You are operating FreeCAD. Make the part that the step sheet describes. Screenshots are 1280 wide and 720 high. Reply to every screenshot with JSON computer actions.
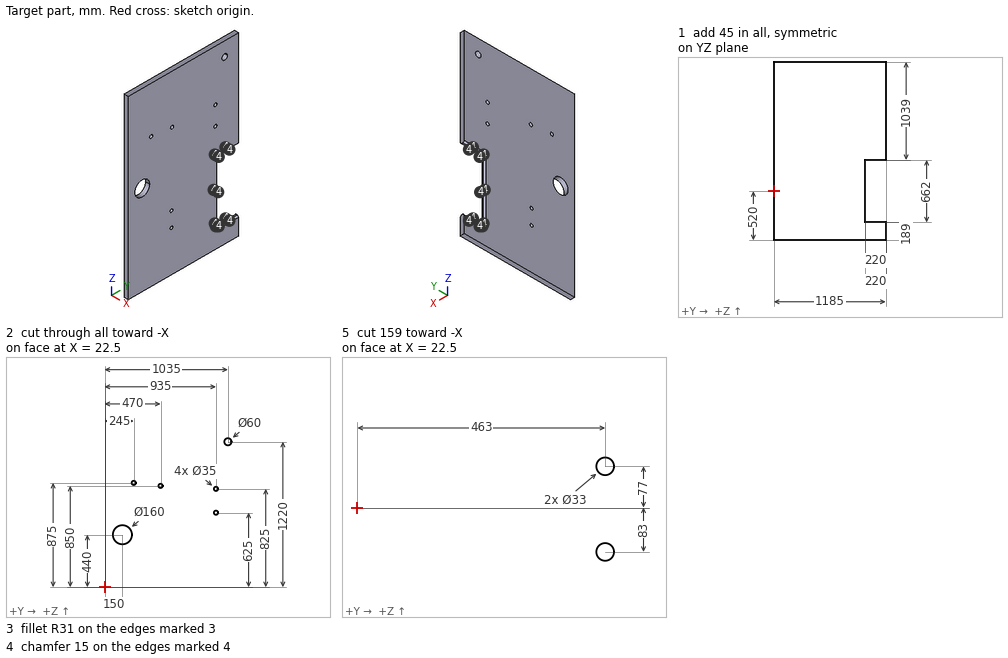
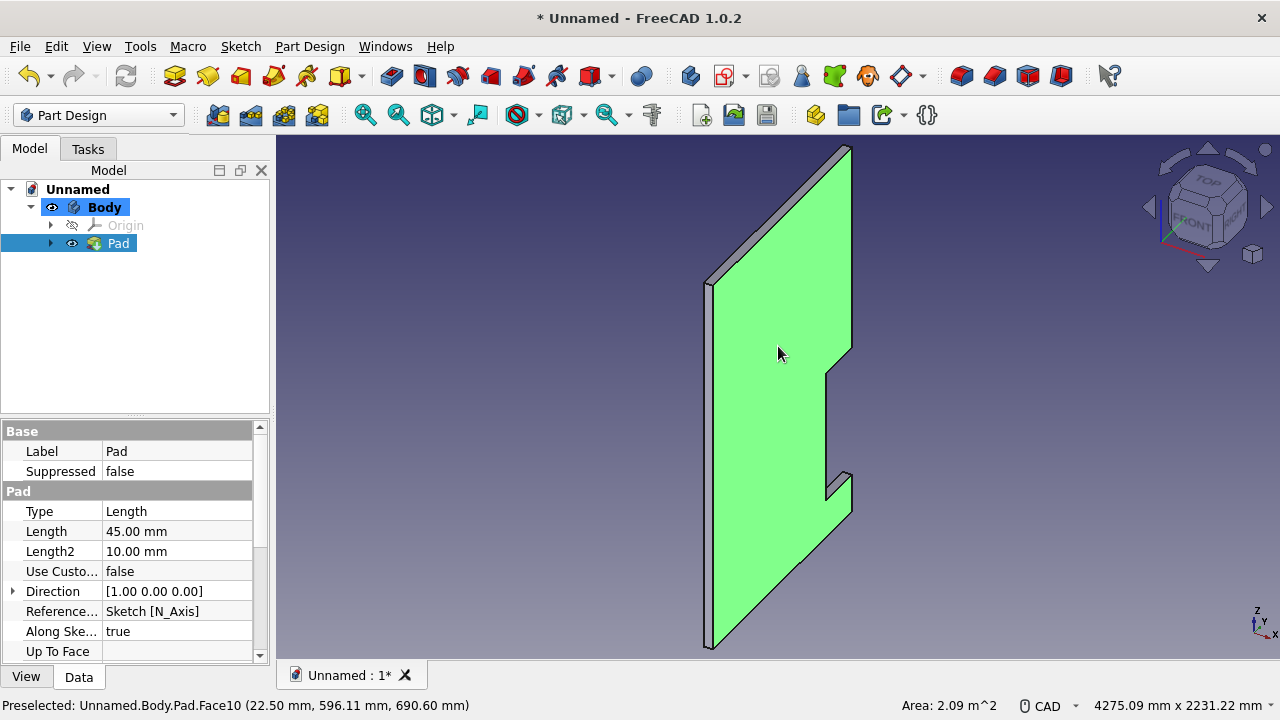
{"action": "left_click", "coordinate": [724, 76]}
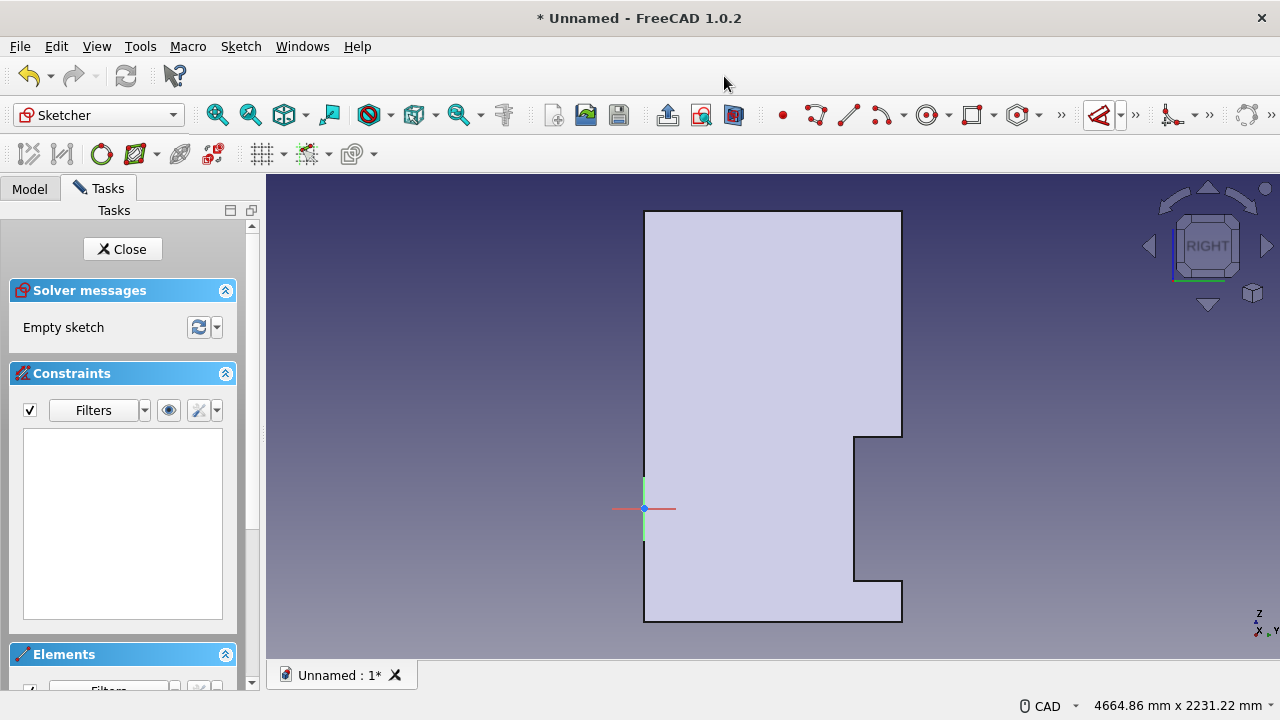
{"action": "left_click", "coordinate": [926, 116]}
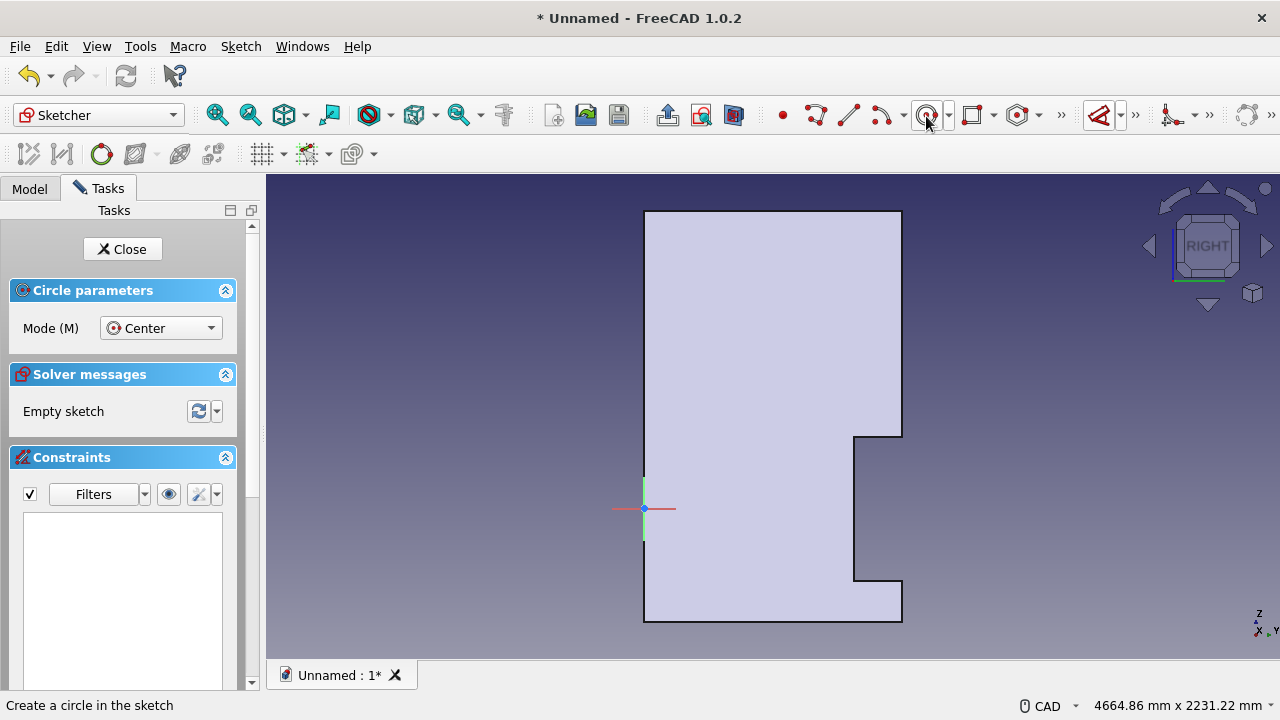
{"action": "scroll", "coordinate": [869, 244], "scroll_direction": "up", "scroll_amount": 7}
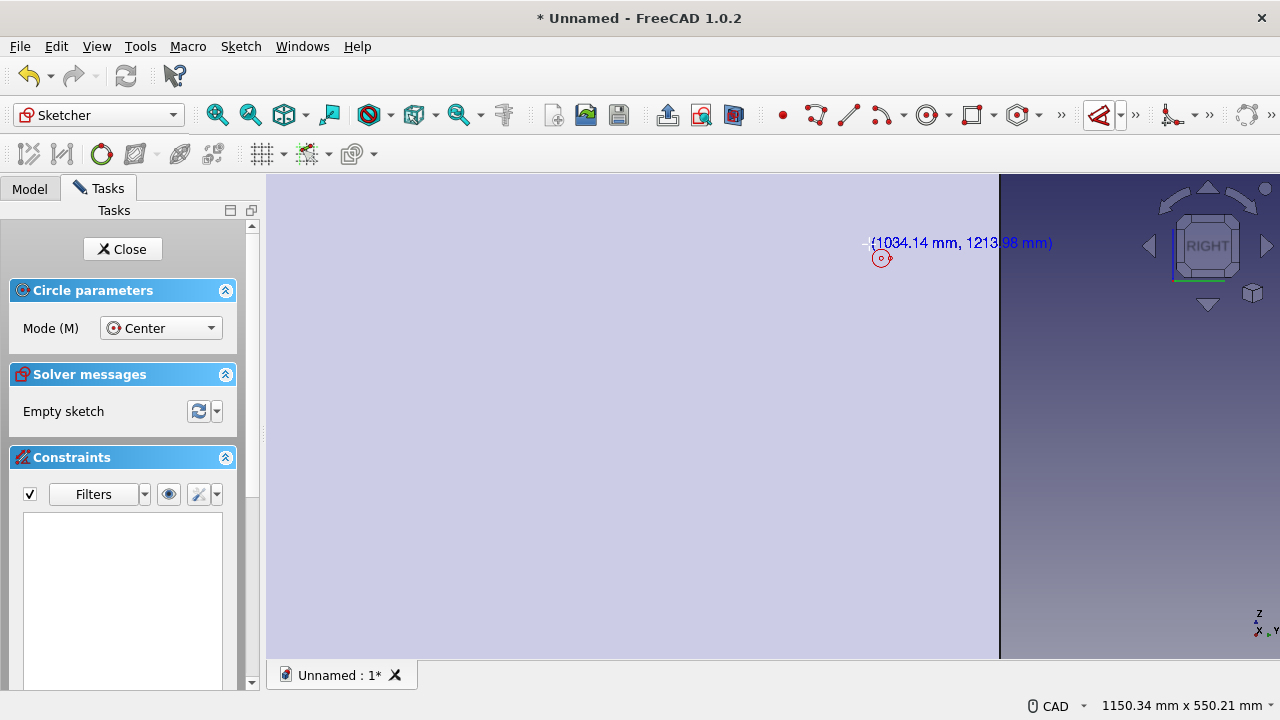
{"action": "scroll", "coordinate": [825, 266], "scroll_direction": "down", "scroll_amount": 6}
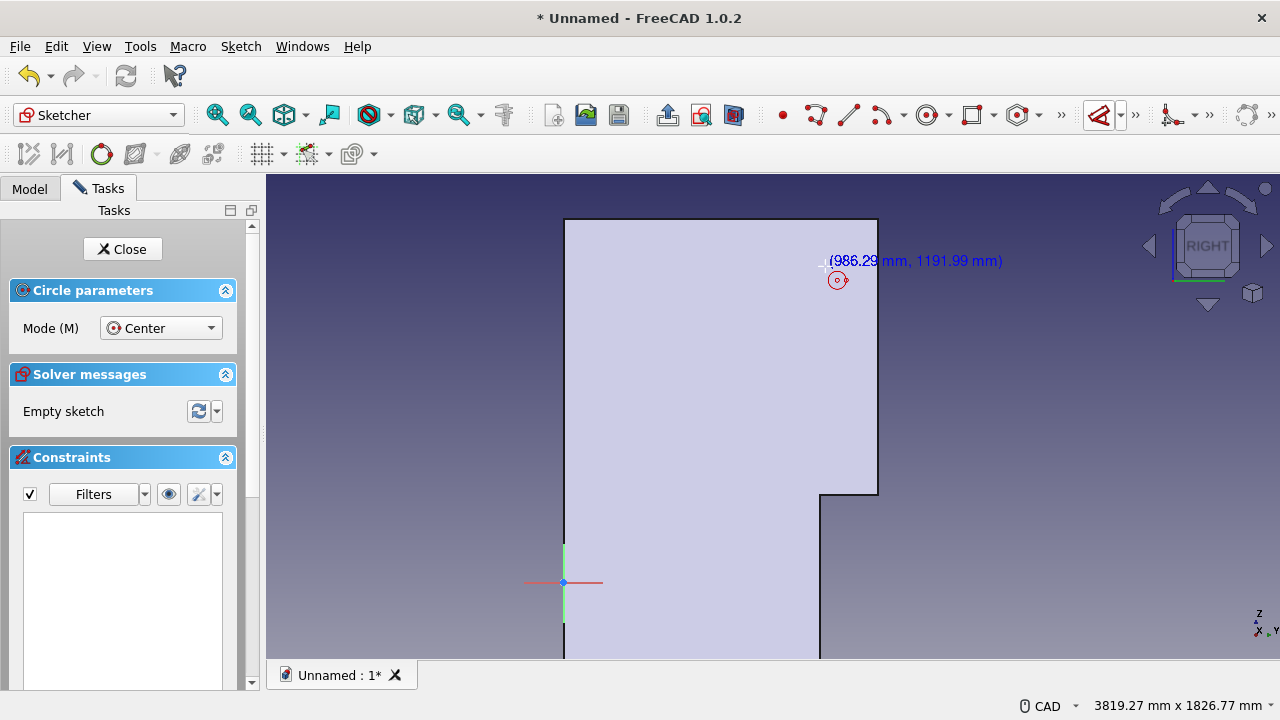
{"action": "left_click", "coordinate": [838, 259]}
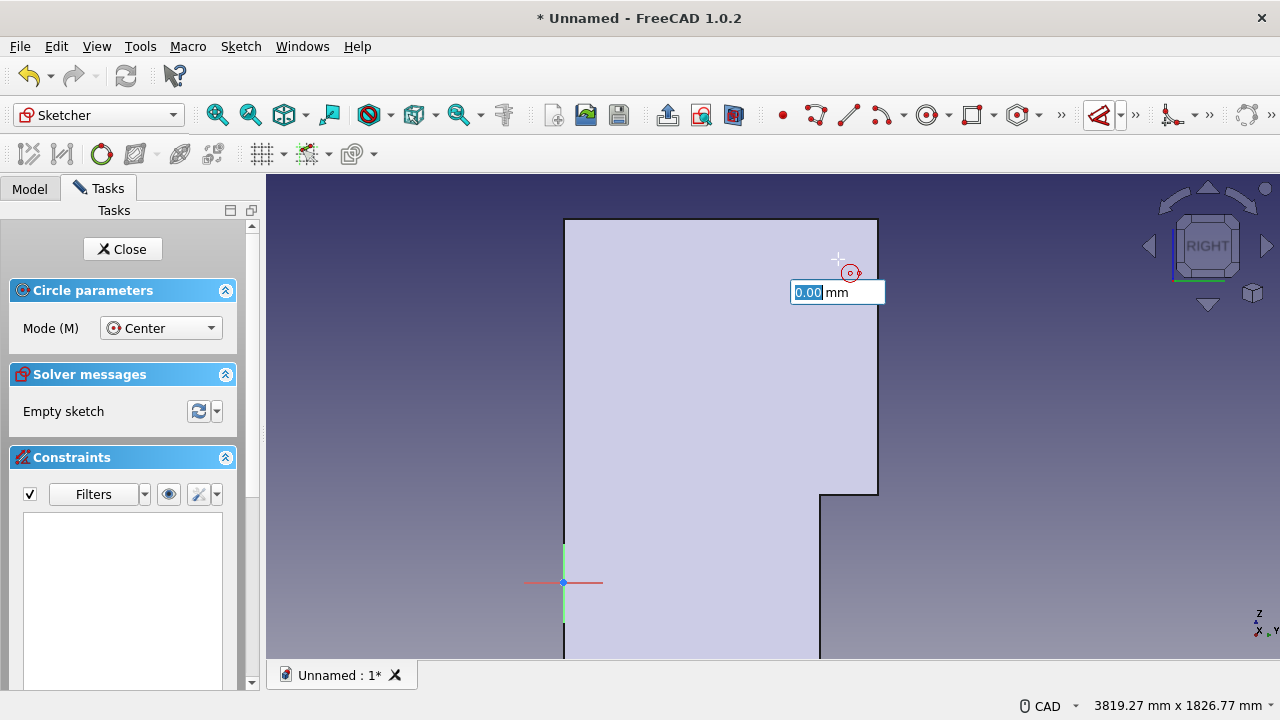
{"action": "scroll", "coordinate": [844, 253], "scroll_direction": "up", "scroll_amount": 4}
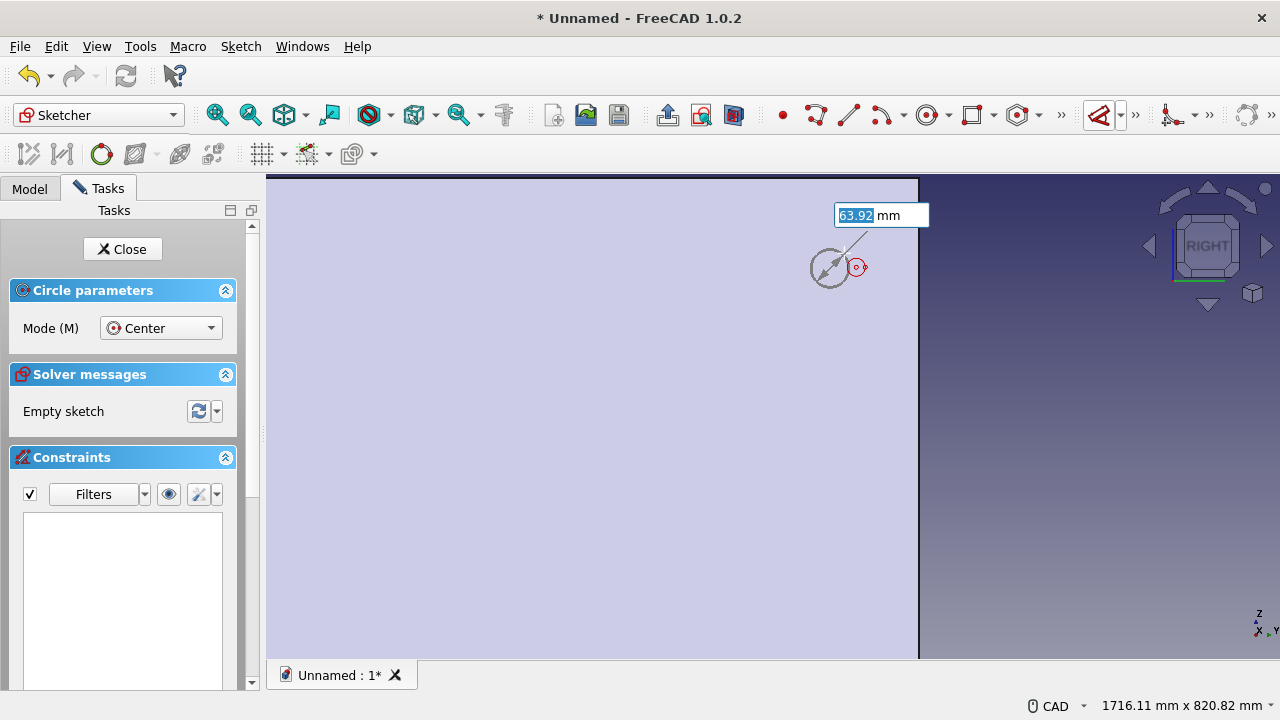
{"action": "left_click", "coordinate": [843, 254]}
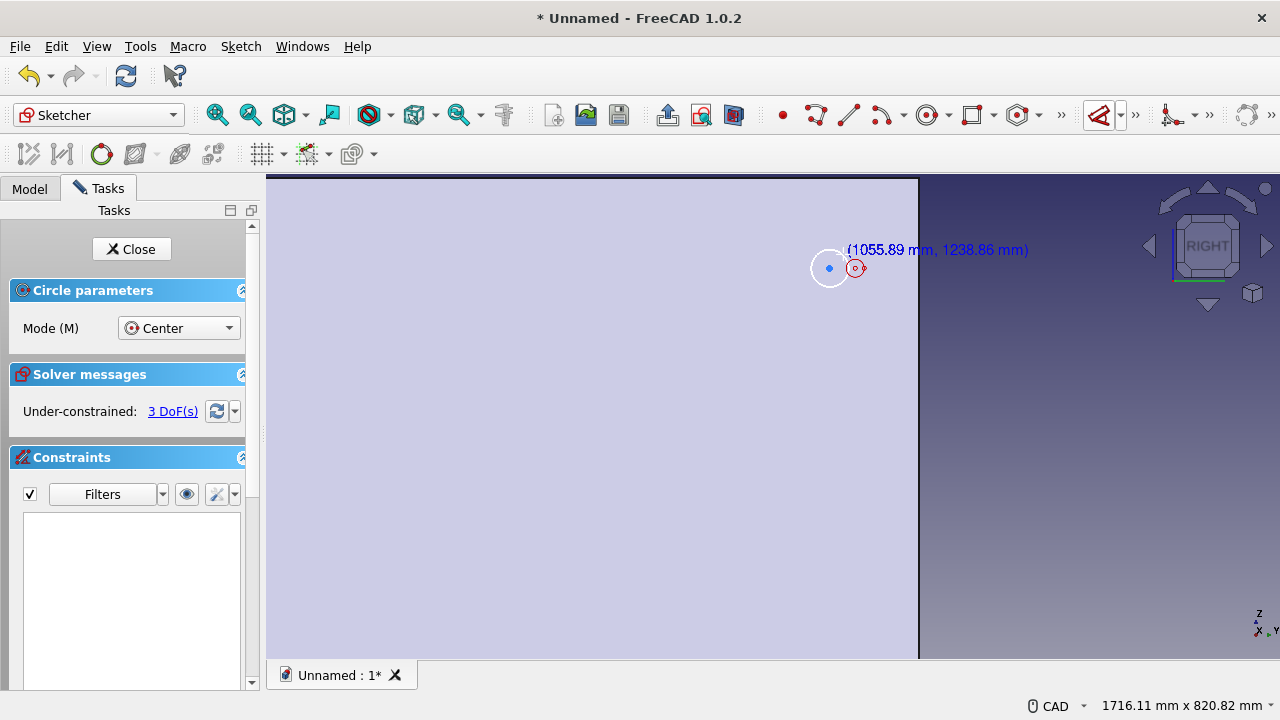
{"action": "scroll", "coordinate": [772, 500], "scroll_direction": "up", "scroll_amount": 4}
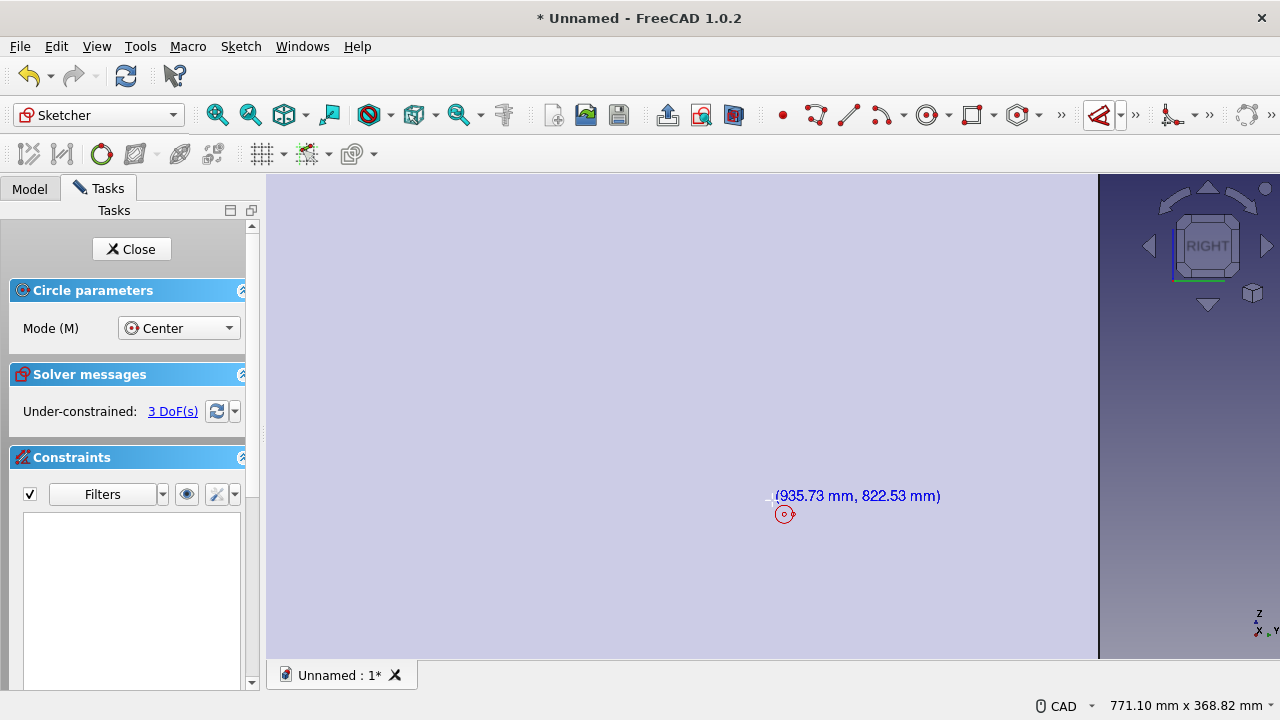
{"action": "scroll", "coordinate": [822, 329], "scroll_direction": "down", "scroll_amount": 8}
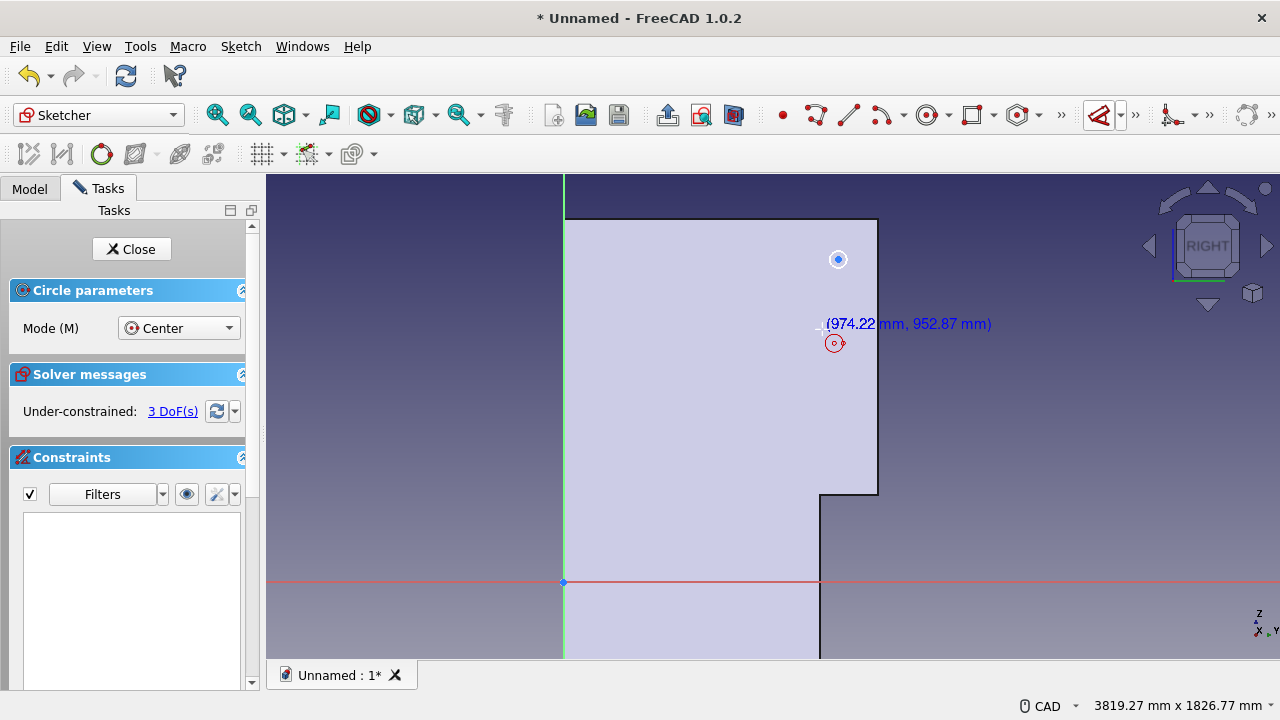
{"action": "left_click", "coordinate": [812, 363]}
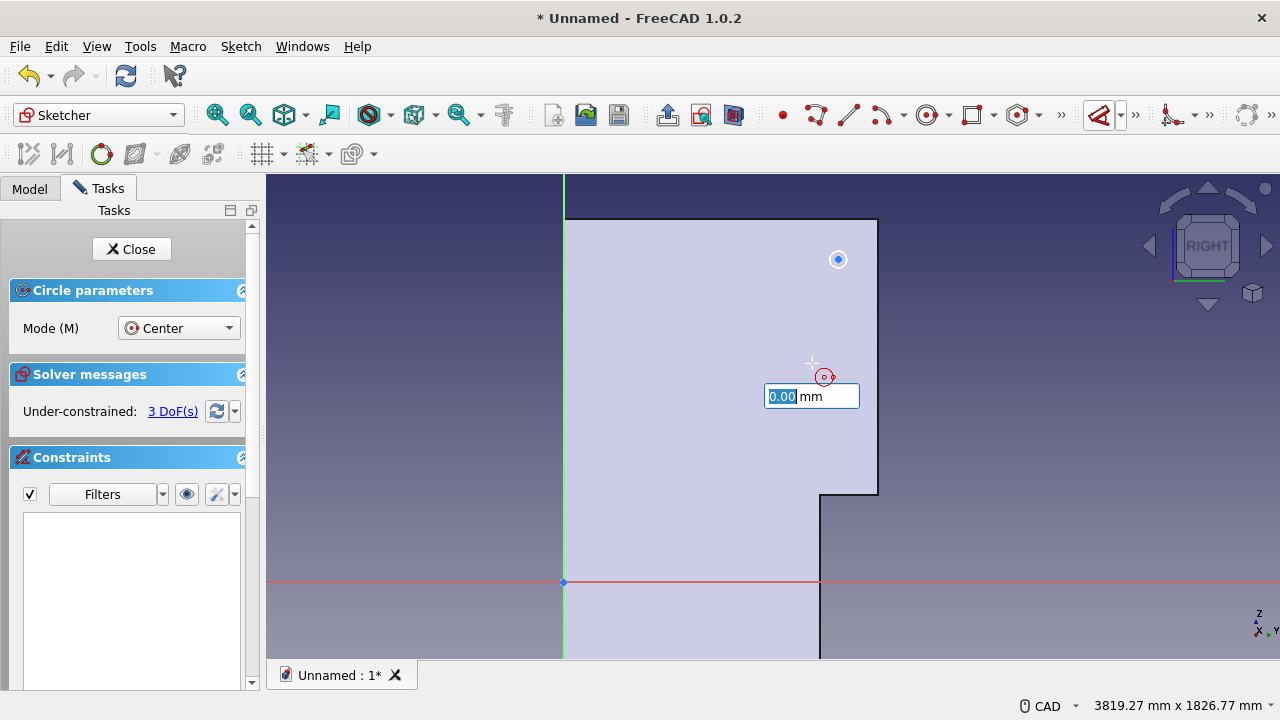
{"action": "scroll", "coordinate": [815, 360], "scroll_direction": "up", "scroll_amount": 7}